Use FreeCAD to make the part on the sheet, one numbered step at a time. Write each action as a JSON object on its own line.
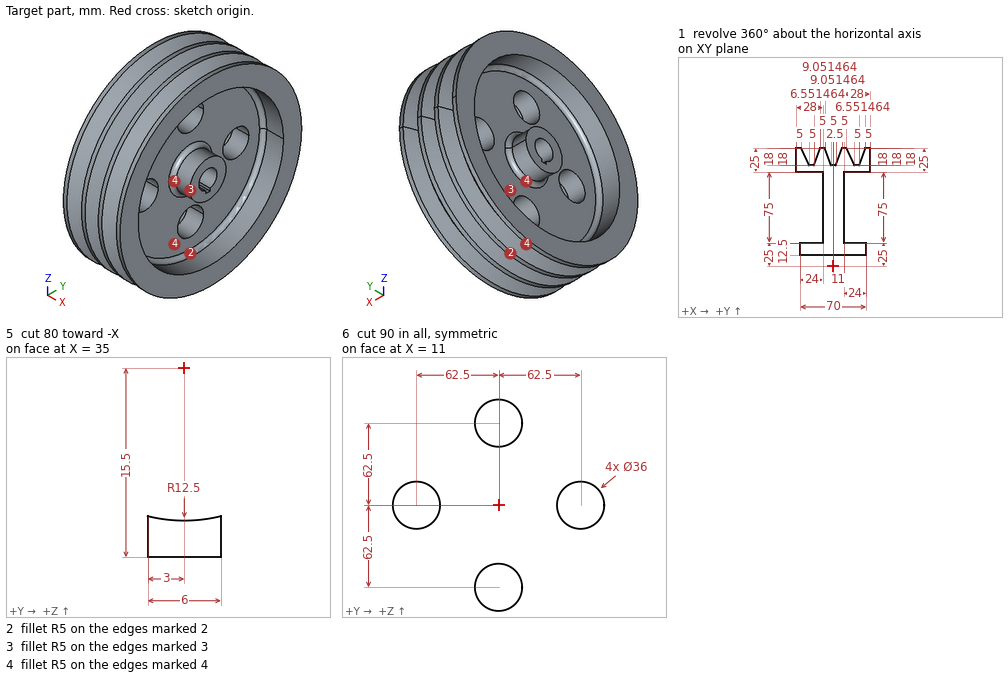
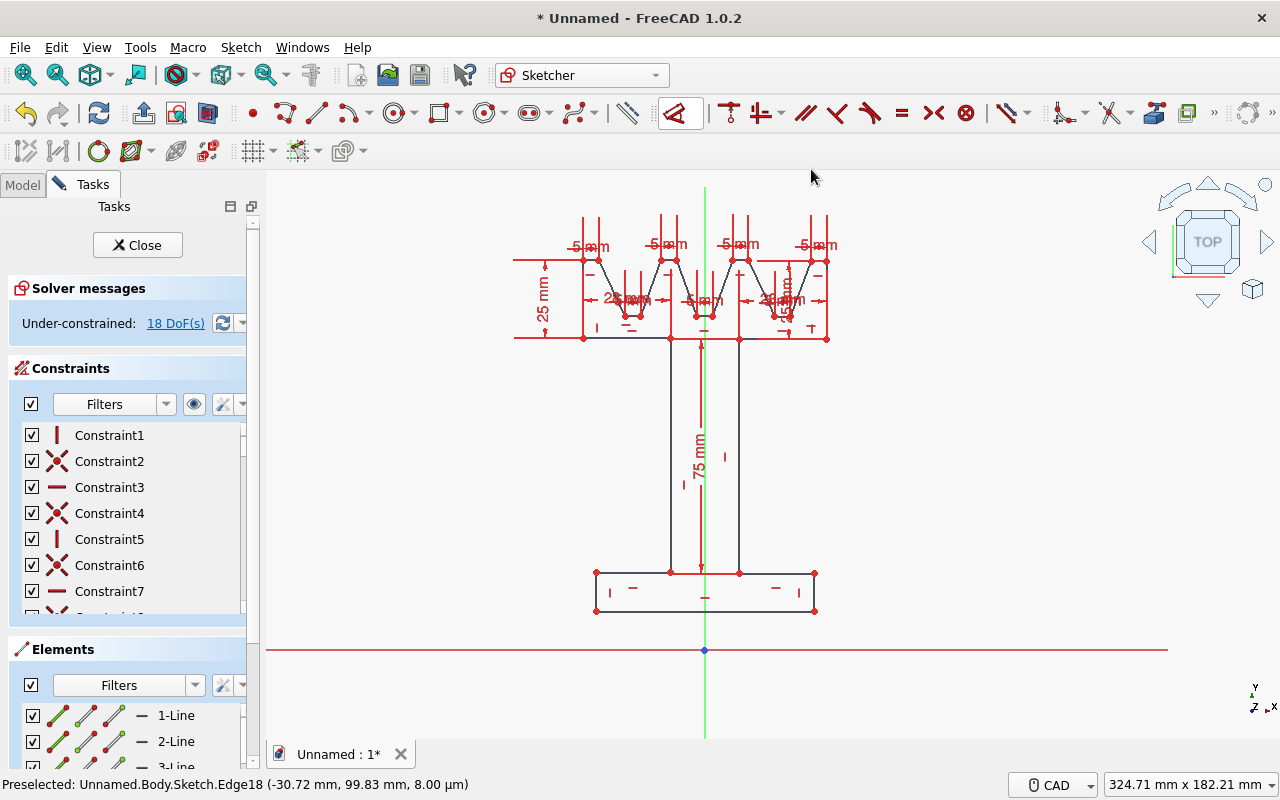
{"action": "left_click", "coordinate": [671, 409]}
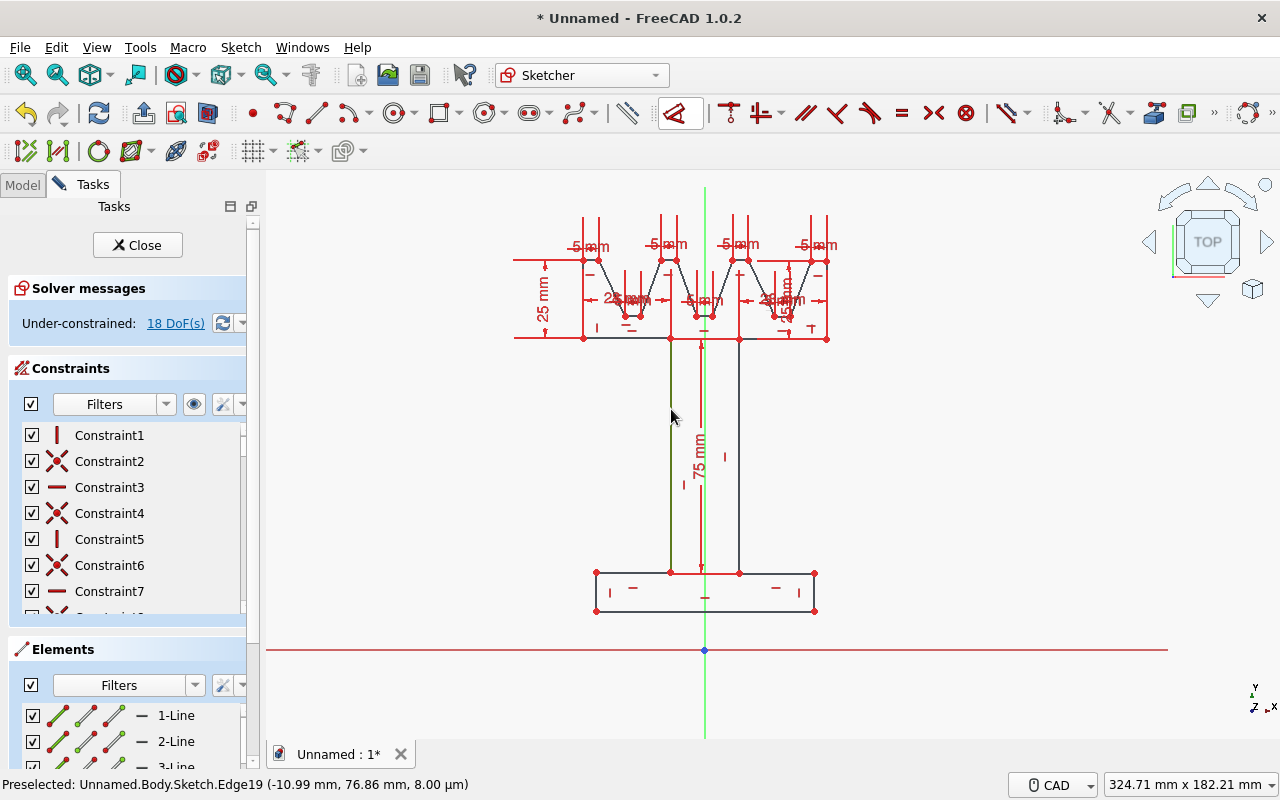
{"action": "left_click", "coordinate": [698, 114]}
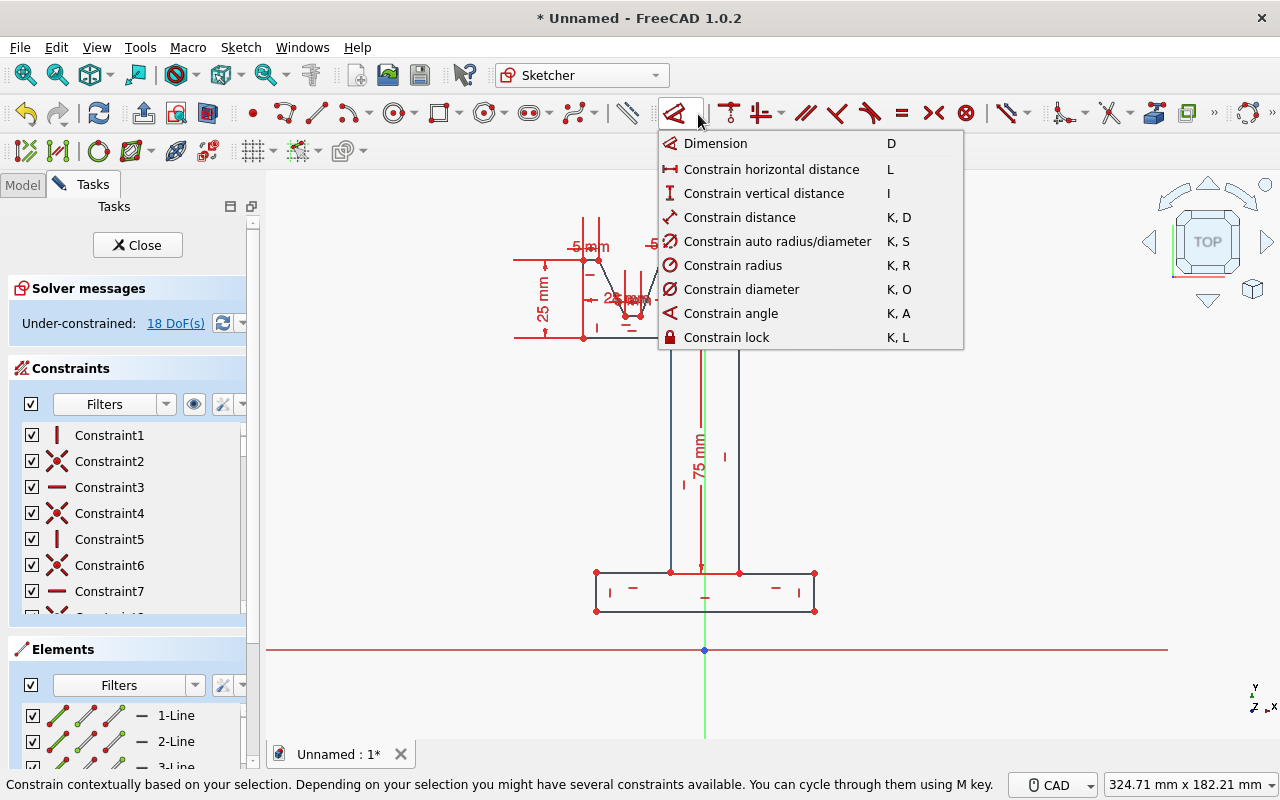
{"action": "left_click", "coordinate": [811, 193]}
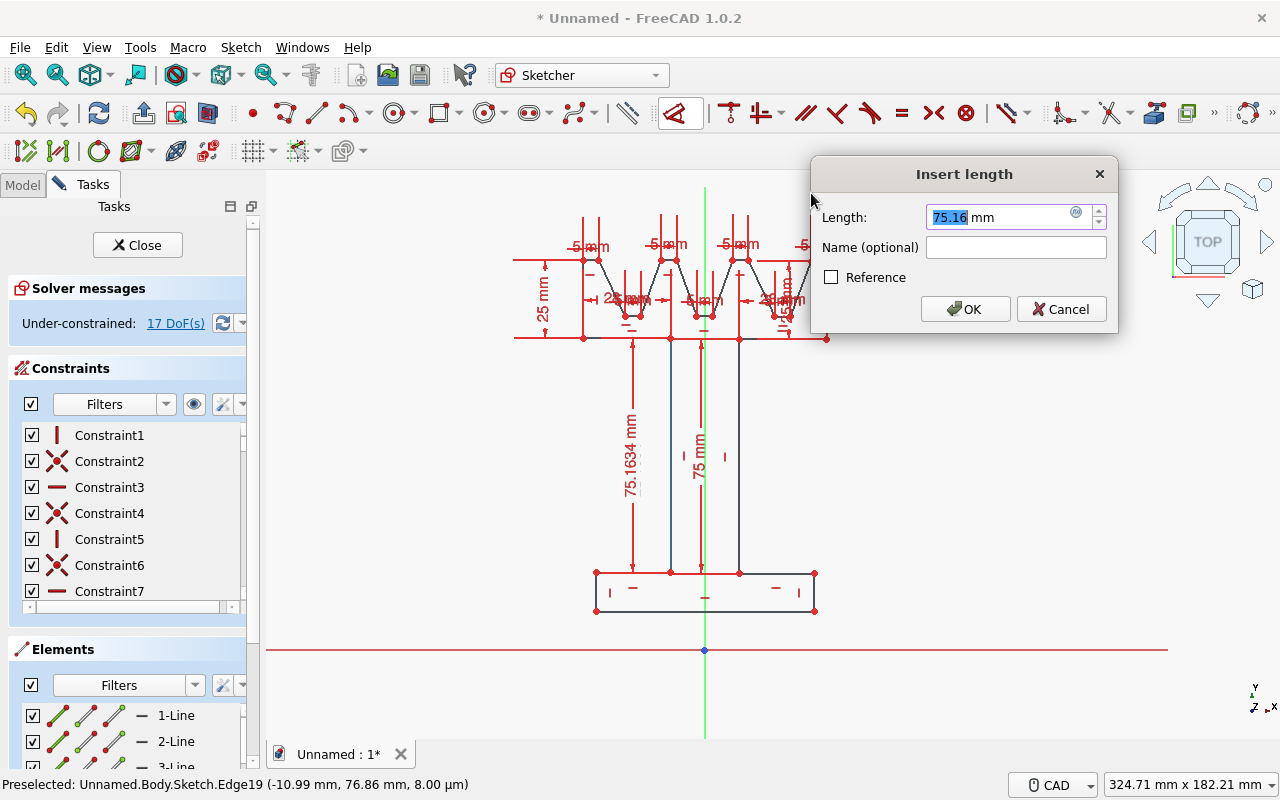
{"action": "type", "text": "75"}
{"action": "key", "text": "Return"}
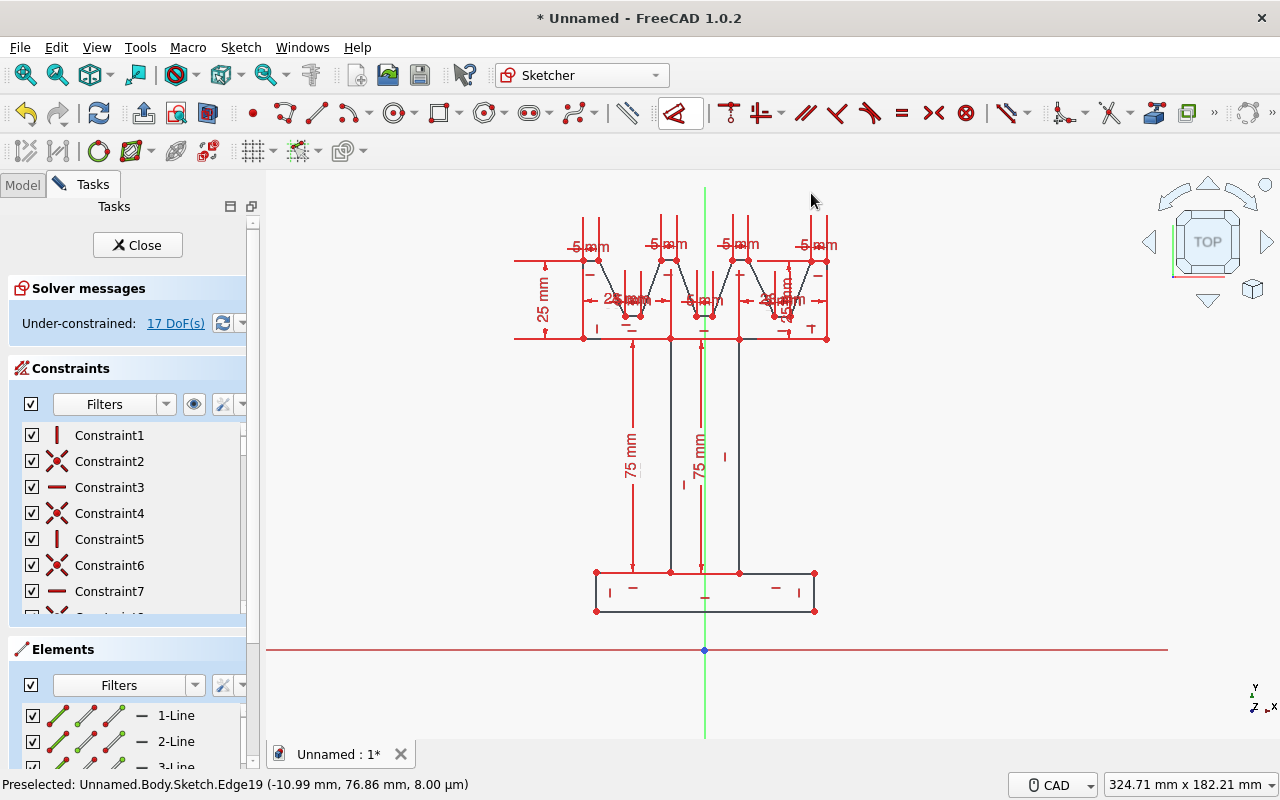
{"action": "left_click", "coordinate": [648, 573]}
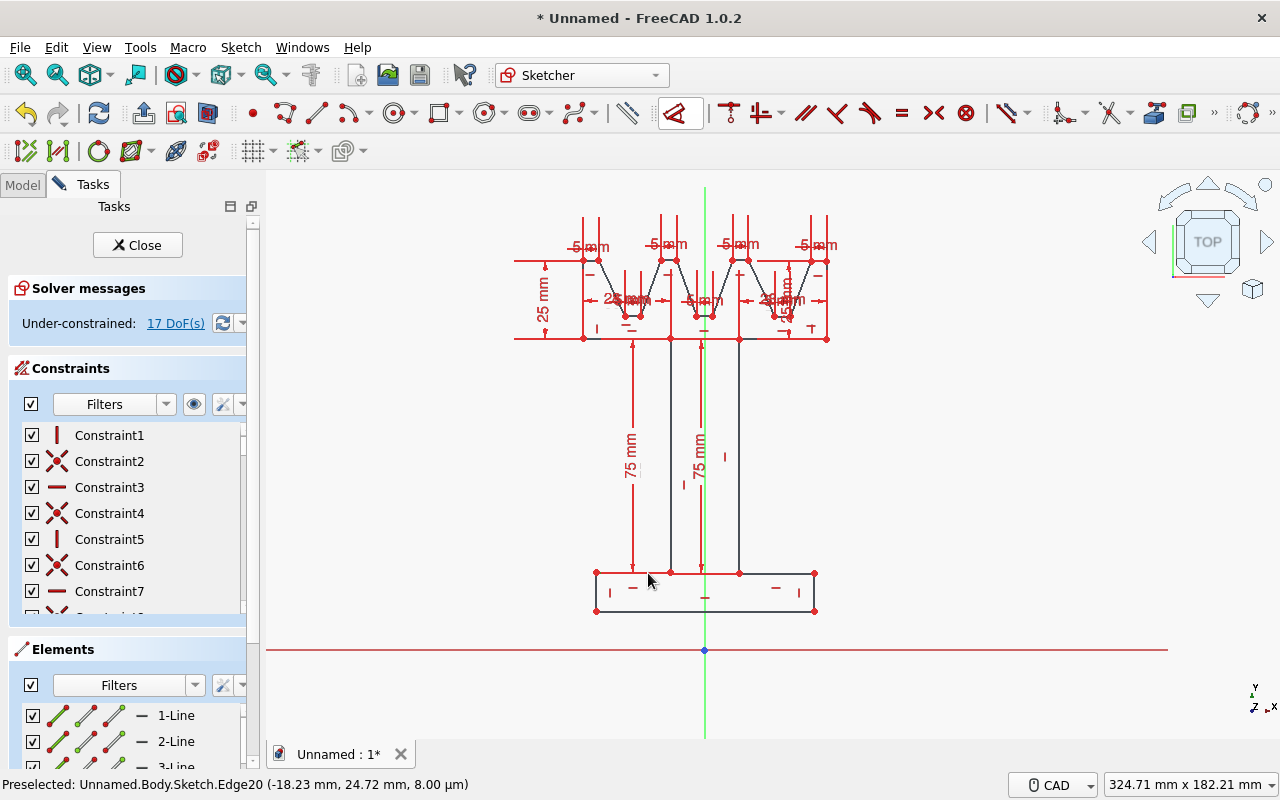
{"action": "left_click", "coordinate": [698, 114]}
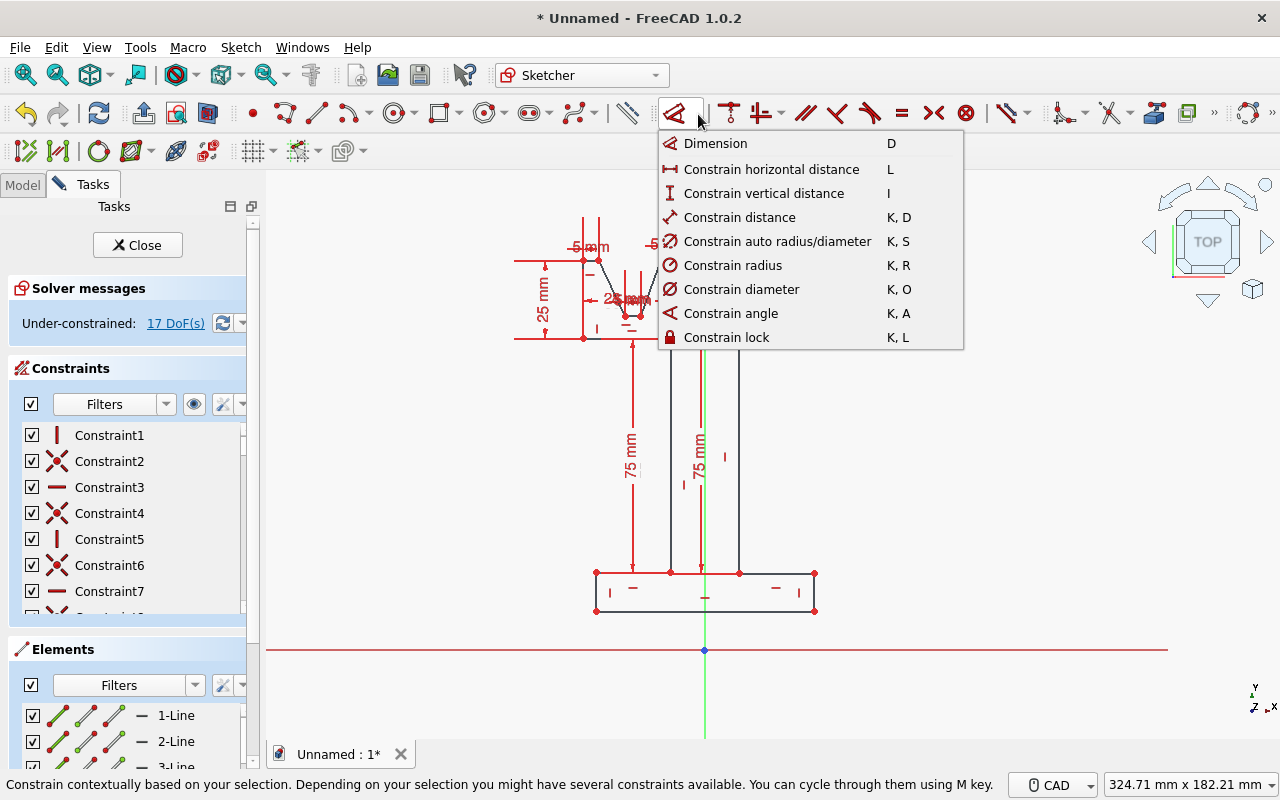
{"action": "left_click", "coordinate": [811, 169]}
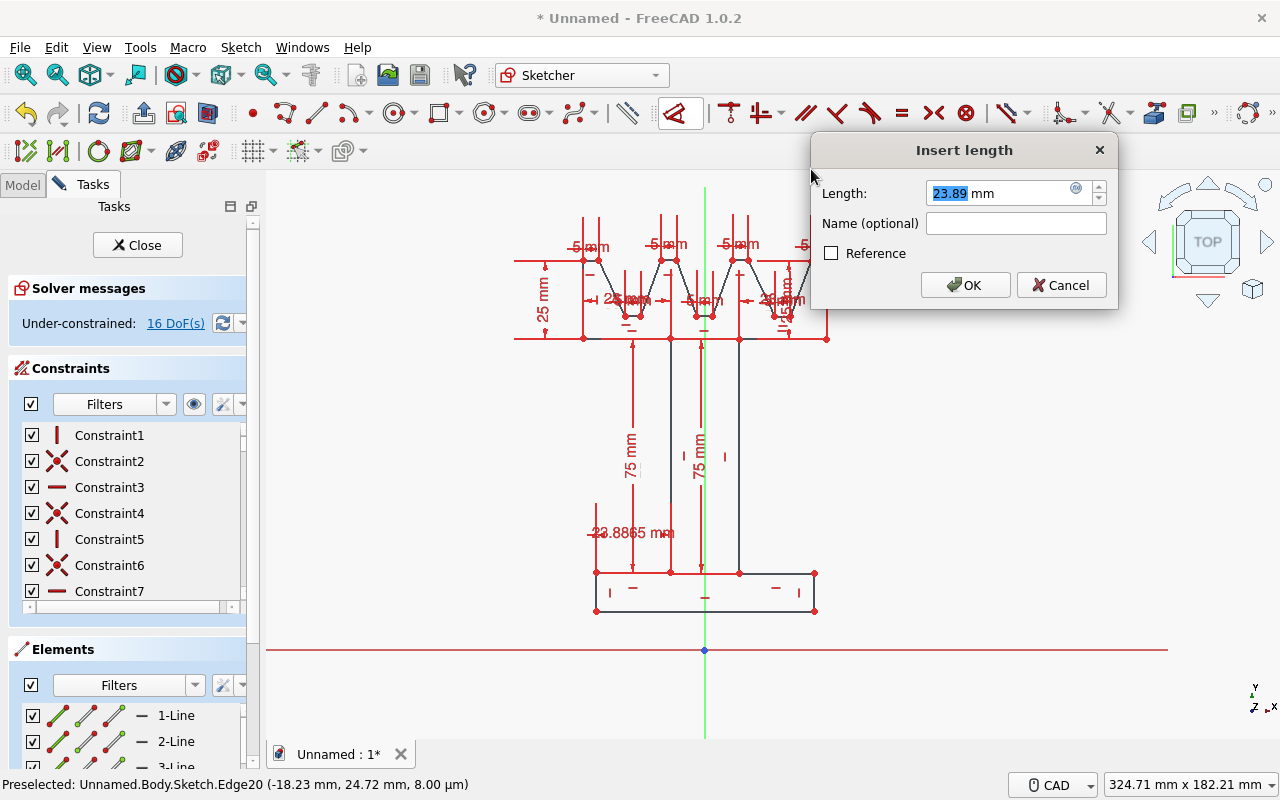
{"action": "type", "text": "24"}
{"action": "key", "text": "Return"}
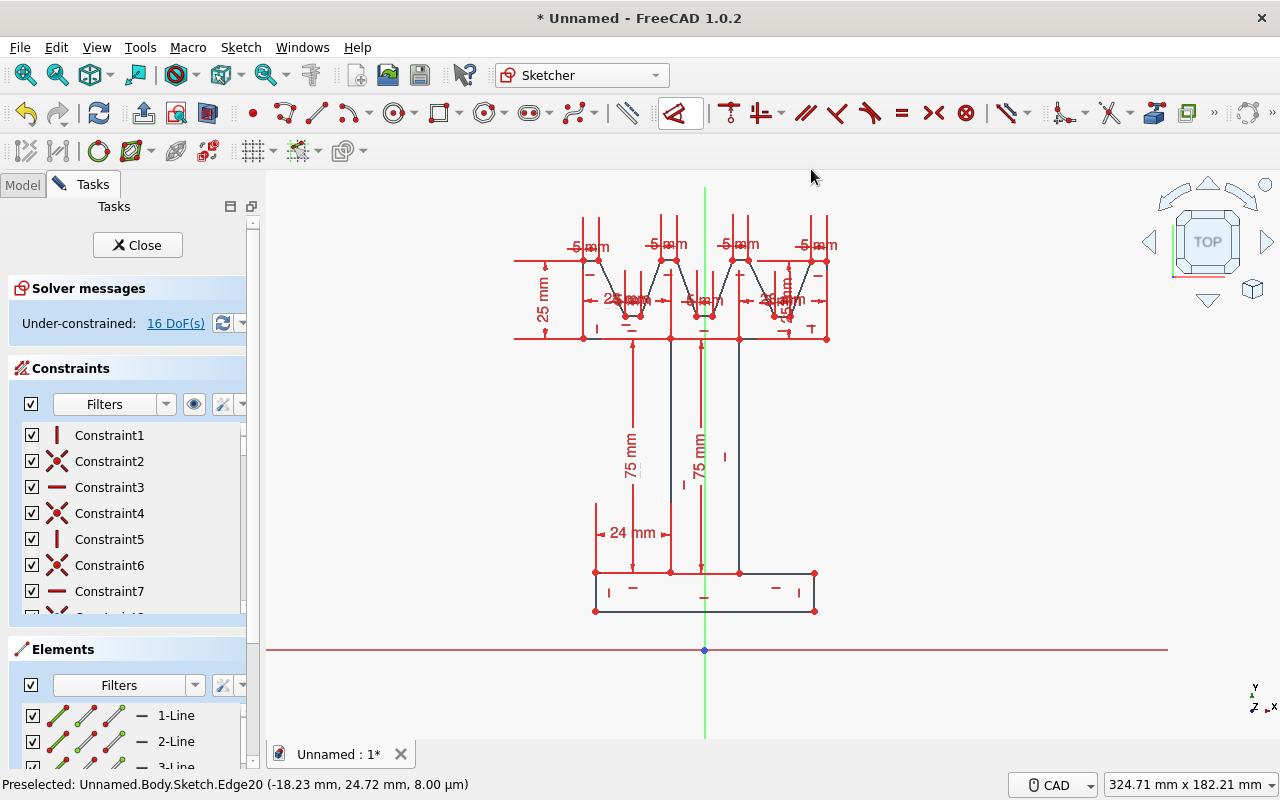
{"action": "left_click", "coordinate": [661, 612]}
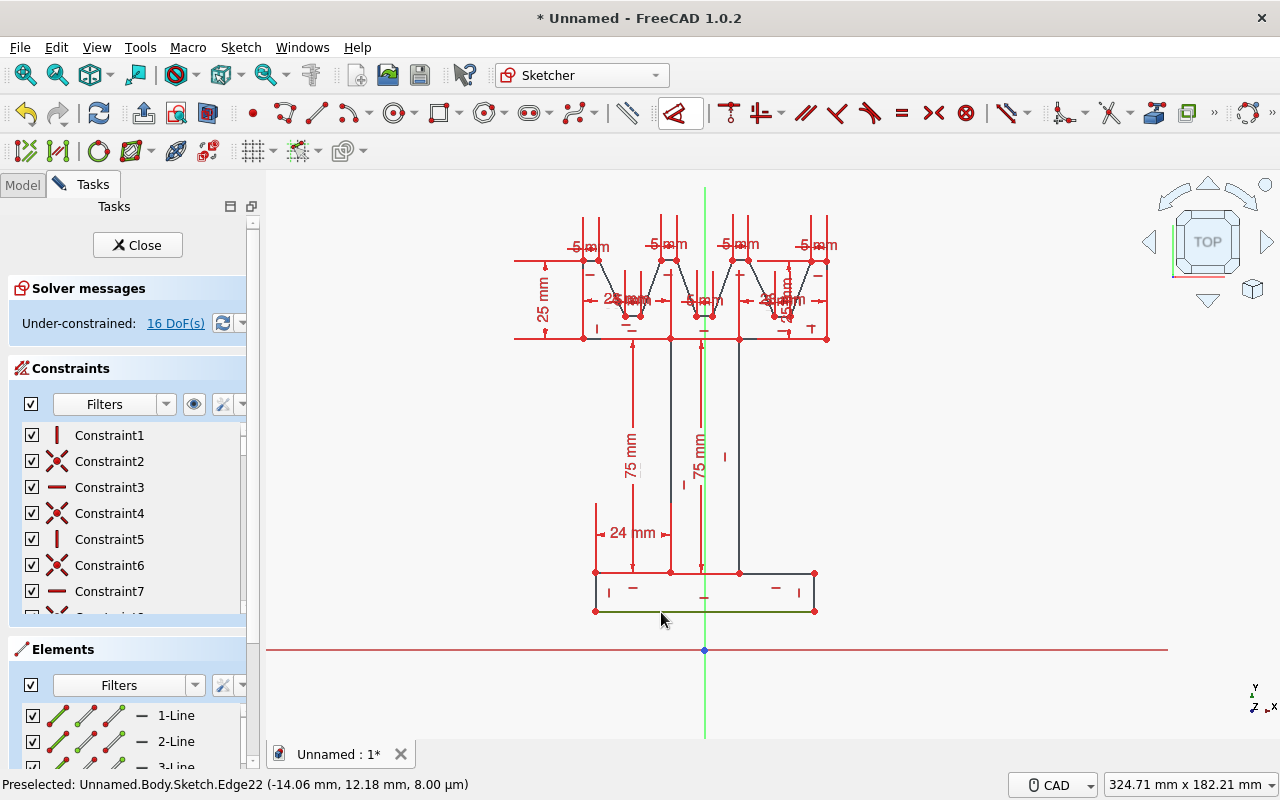
{"action": "key", "text": "l"}